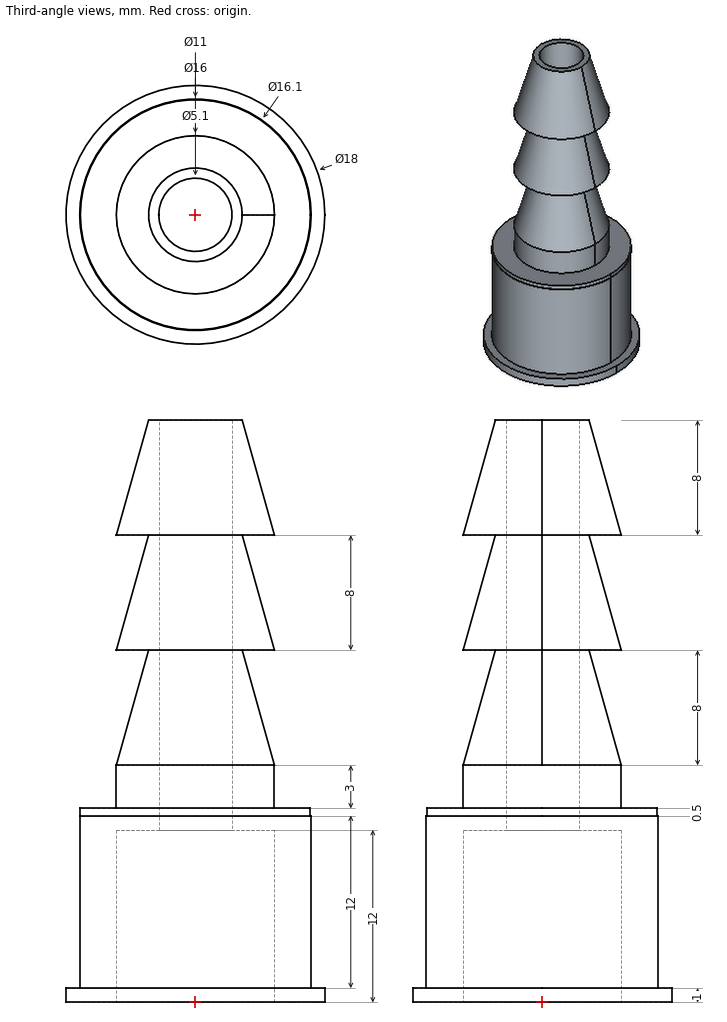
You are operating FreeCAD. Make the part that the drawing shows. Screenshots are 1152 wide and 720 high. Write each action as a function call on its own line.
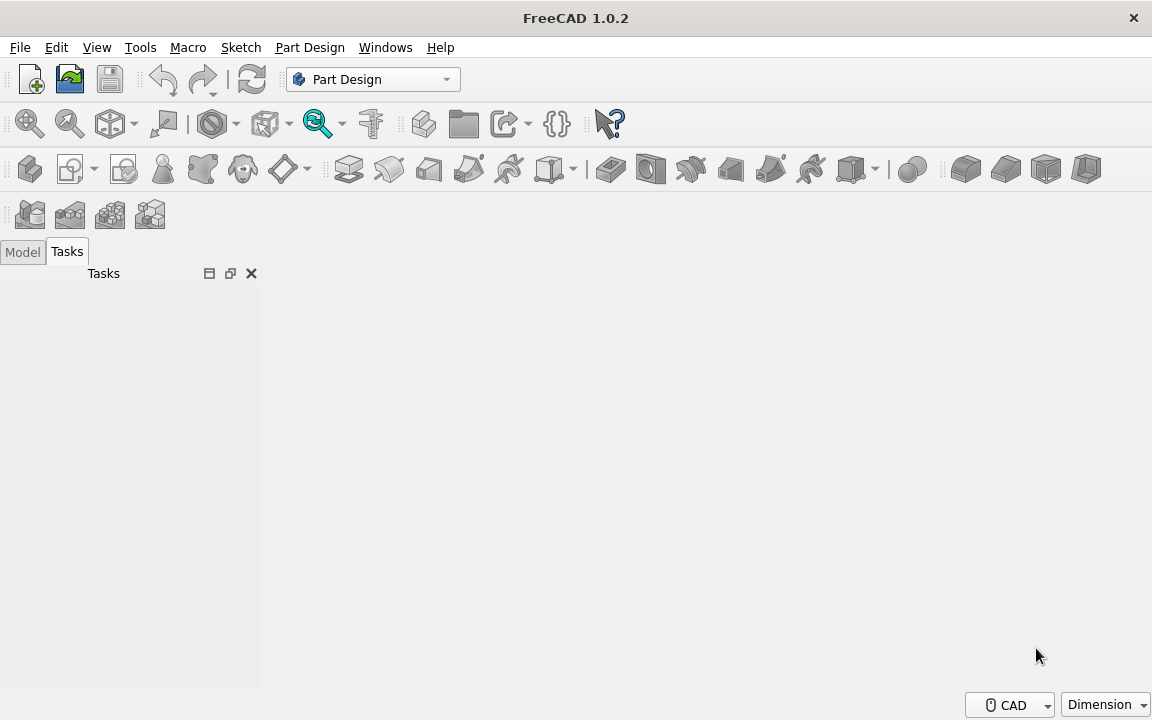
key(ctrl+n)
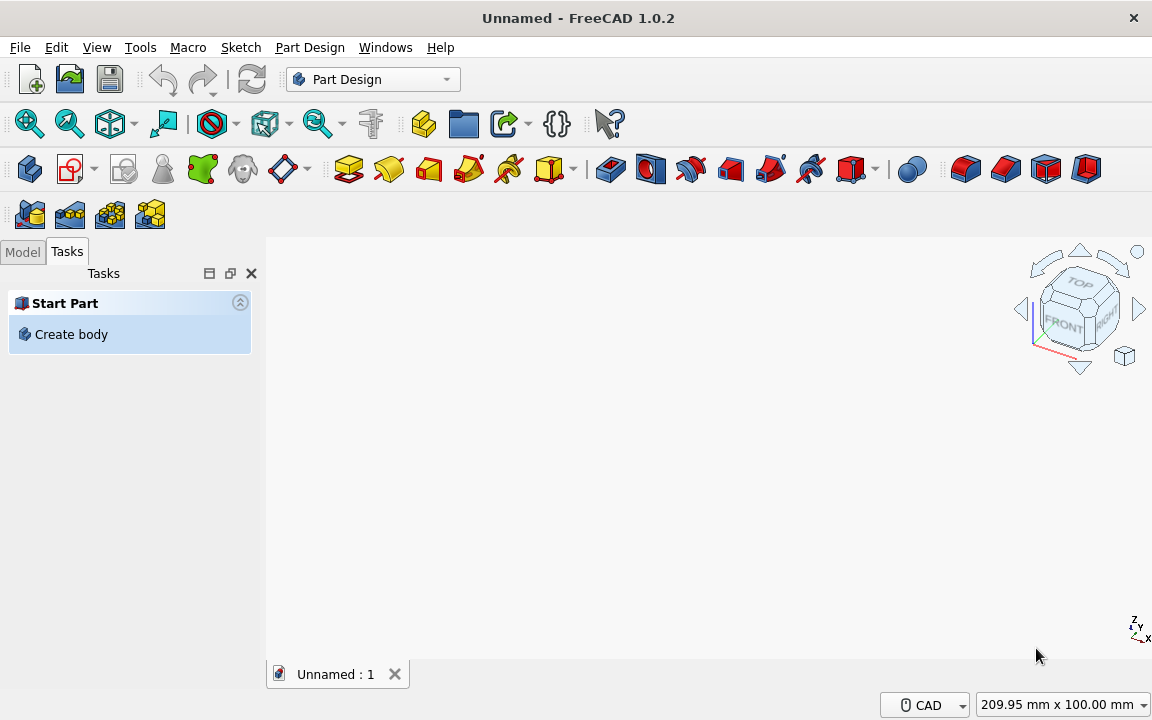
click(70, 170)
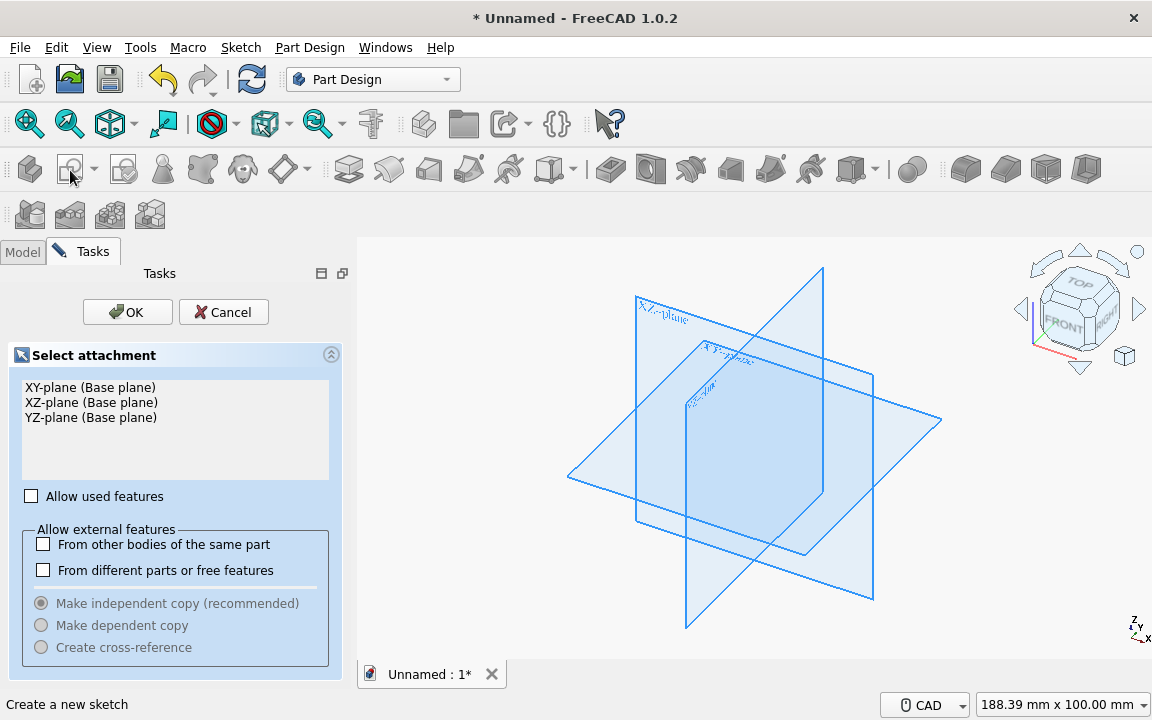
click(82, 388)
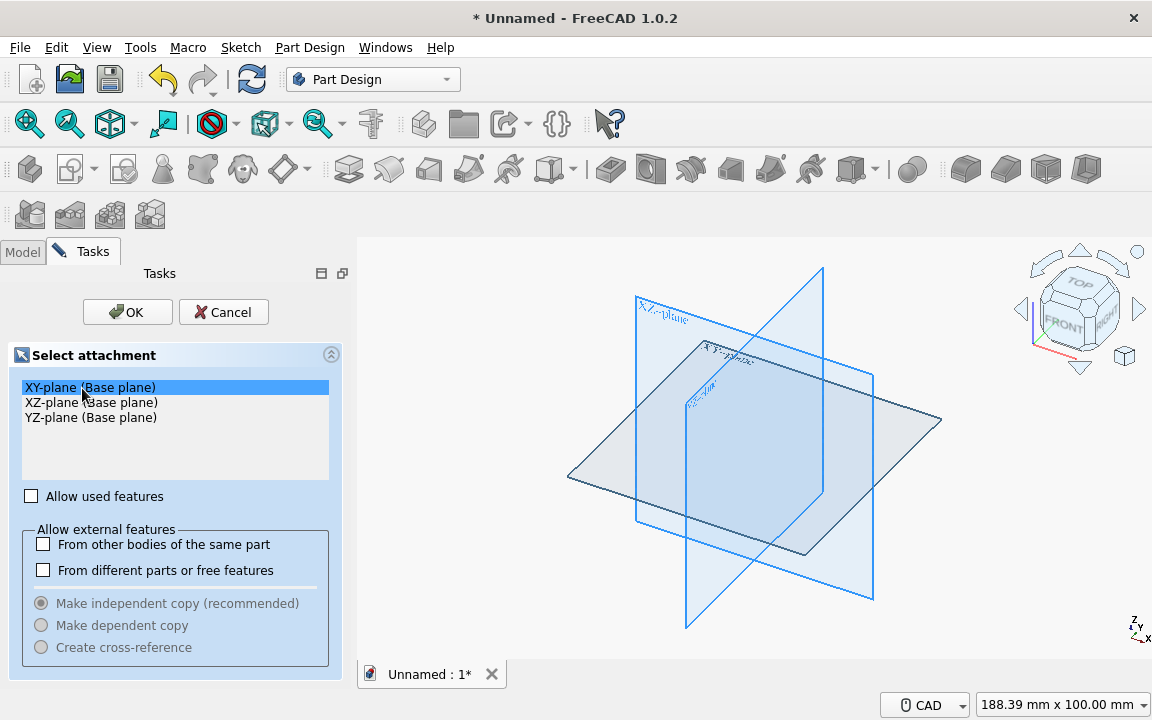
click(128, 312)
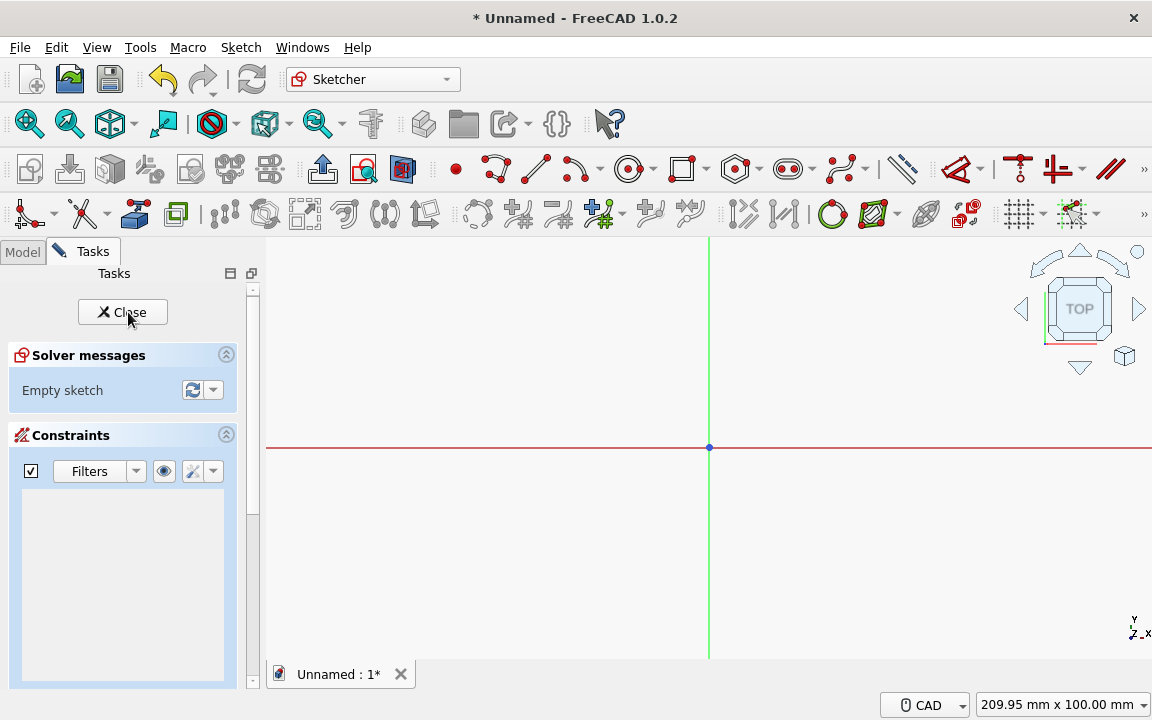
scroll(739, 448, up, 6)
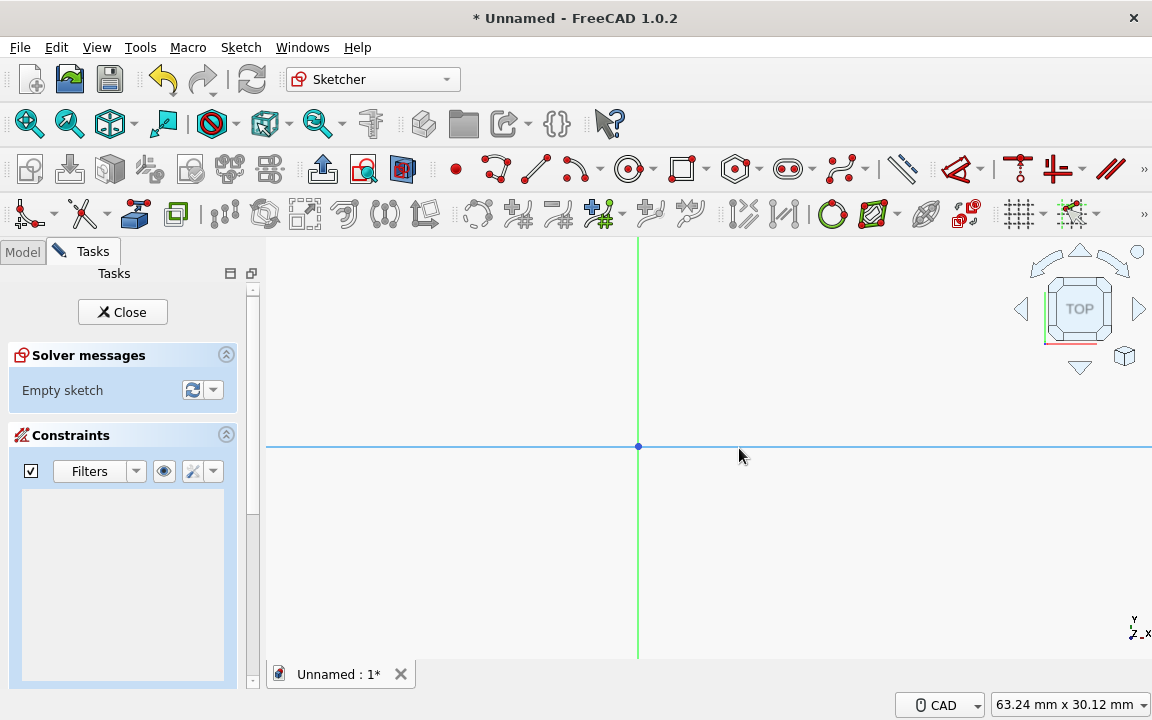
key(g)
key(c)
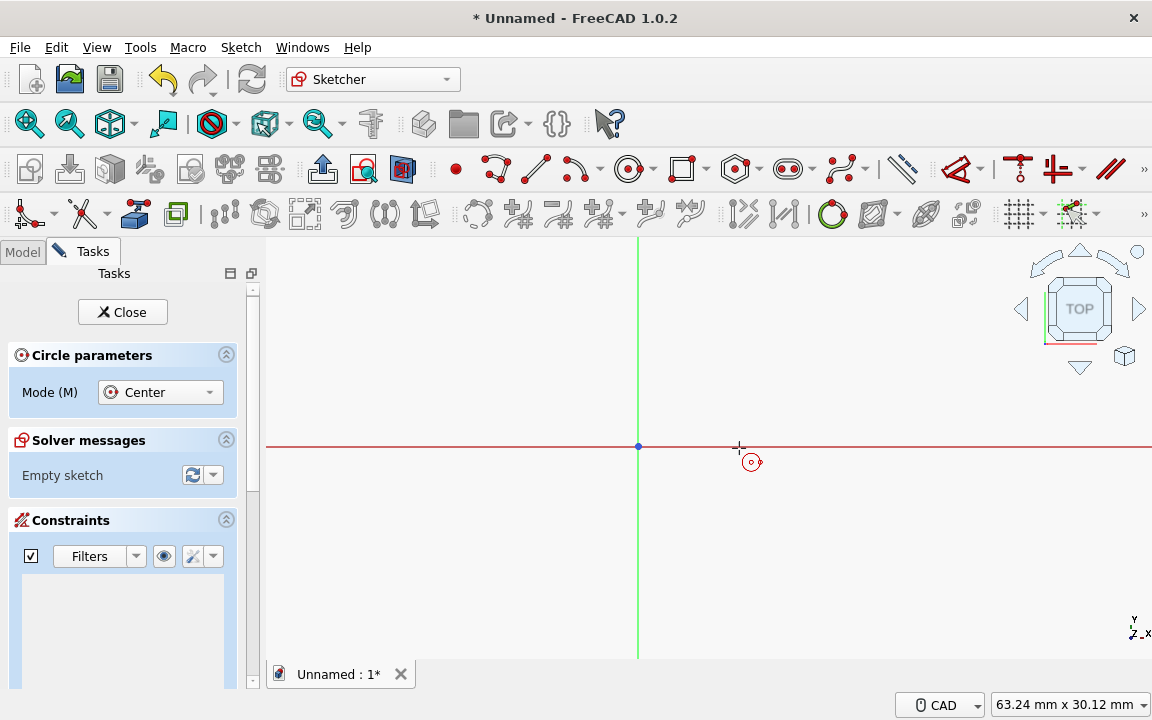
click(638, 447)
click(727, 358)
key(Escape)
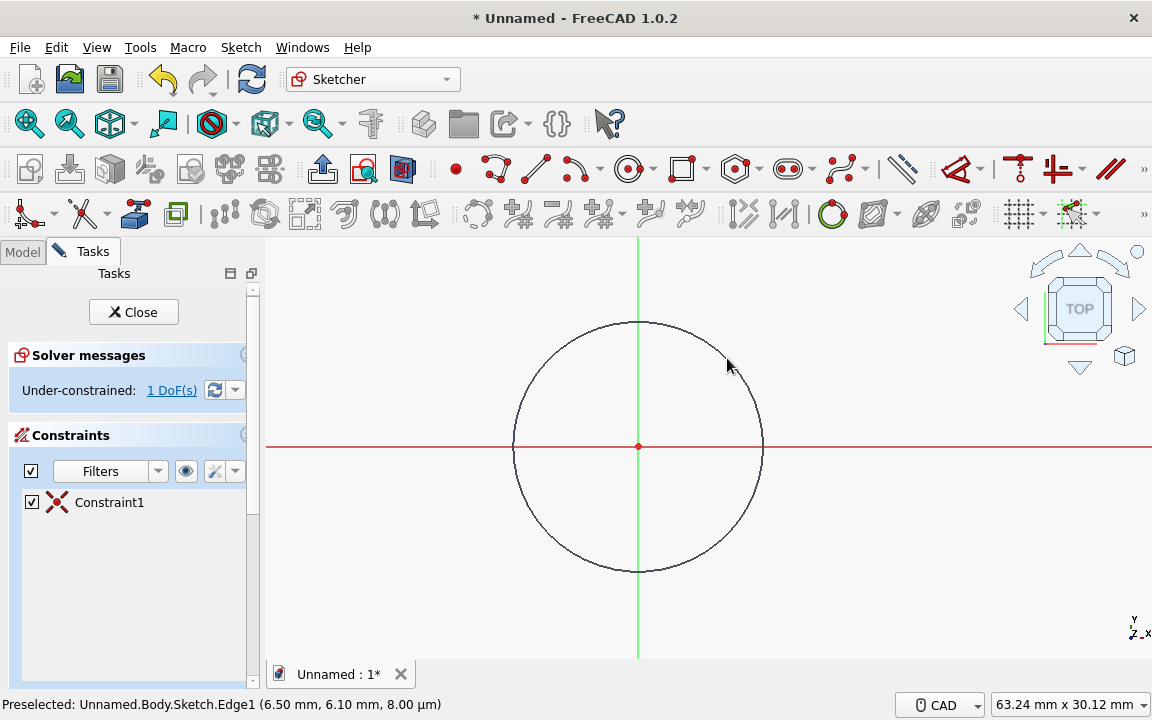
key(d)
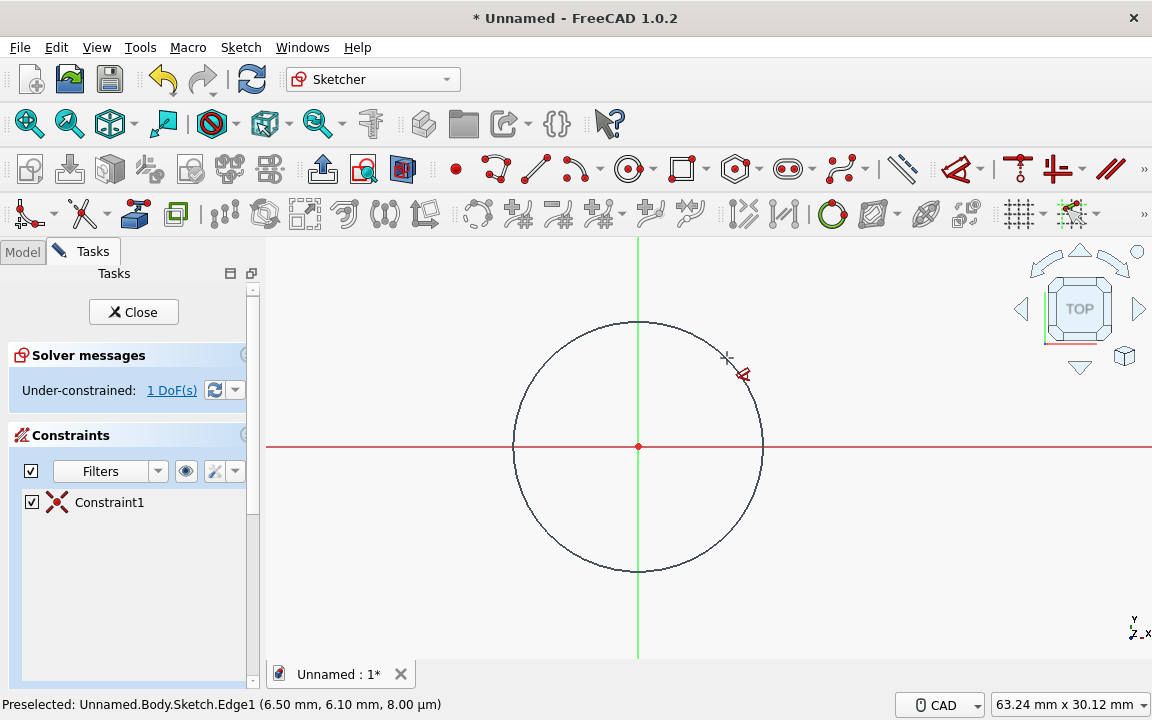
click(726, 358)
click(748, 335)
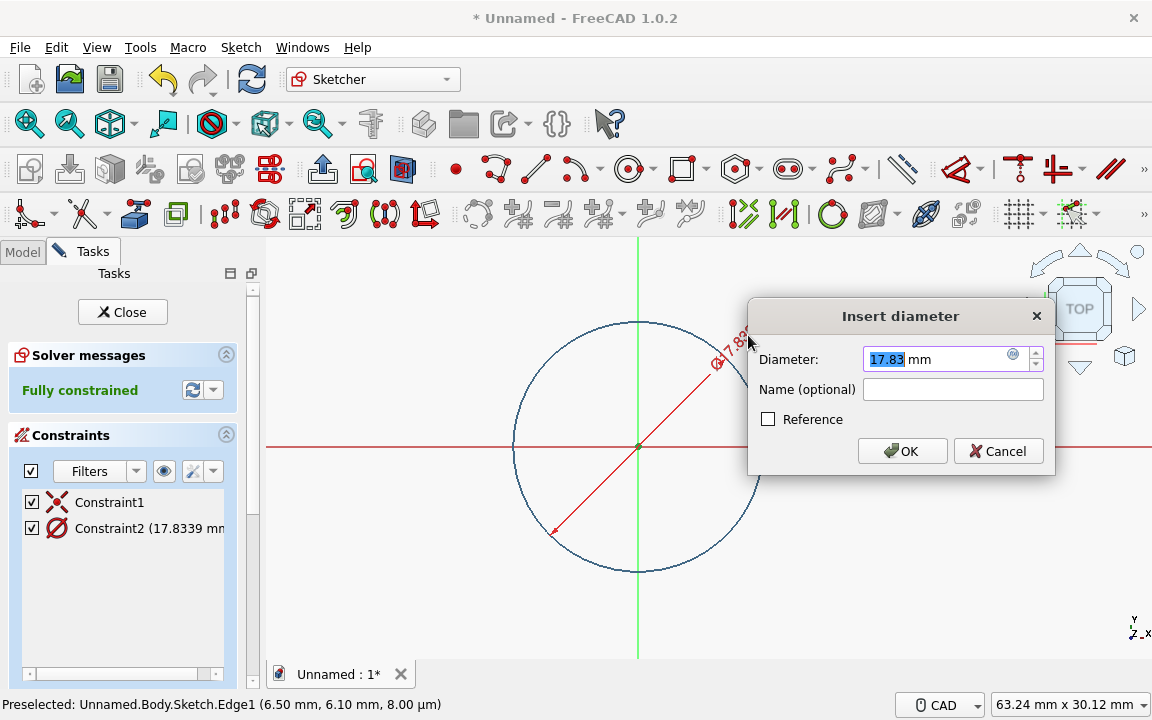
text(18)
key(Return)
key(Escape)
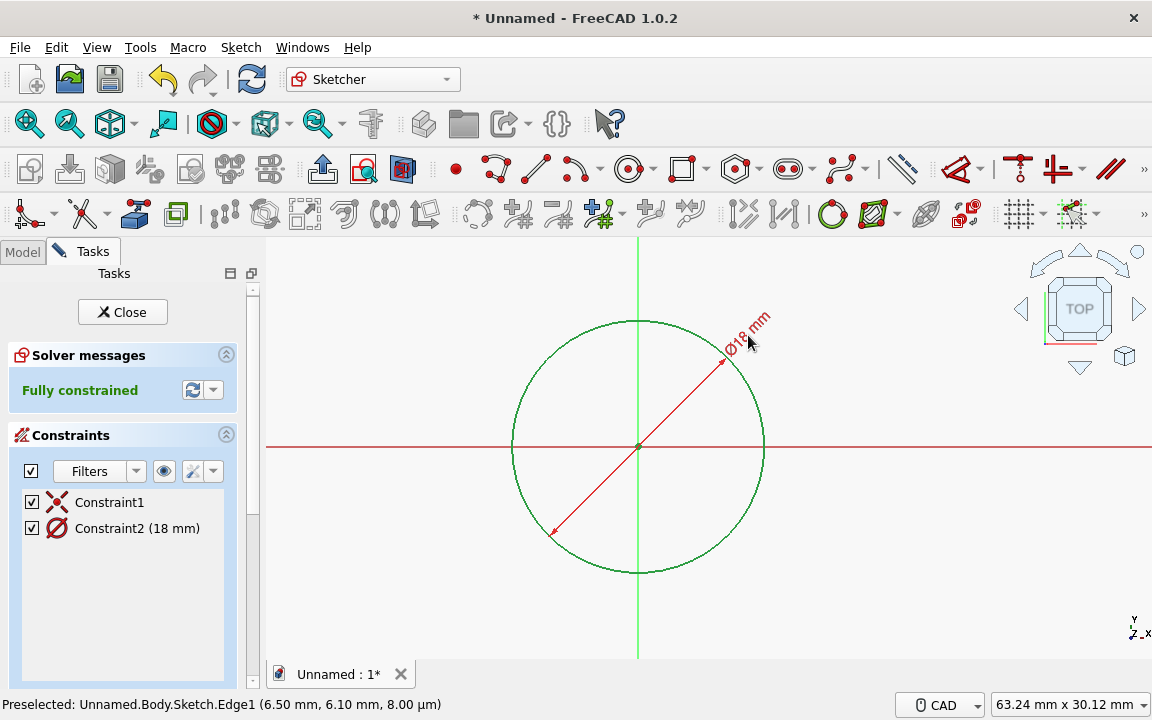
click(123, 312)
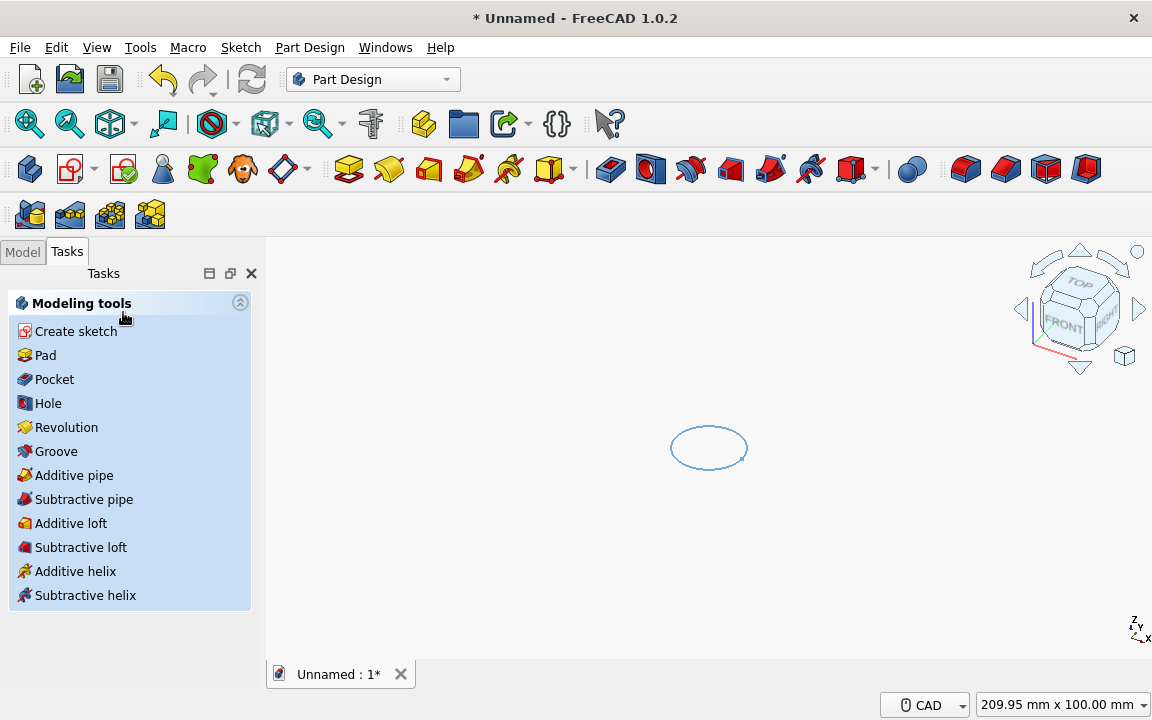
click(350, 170)